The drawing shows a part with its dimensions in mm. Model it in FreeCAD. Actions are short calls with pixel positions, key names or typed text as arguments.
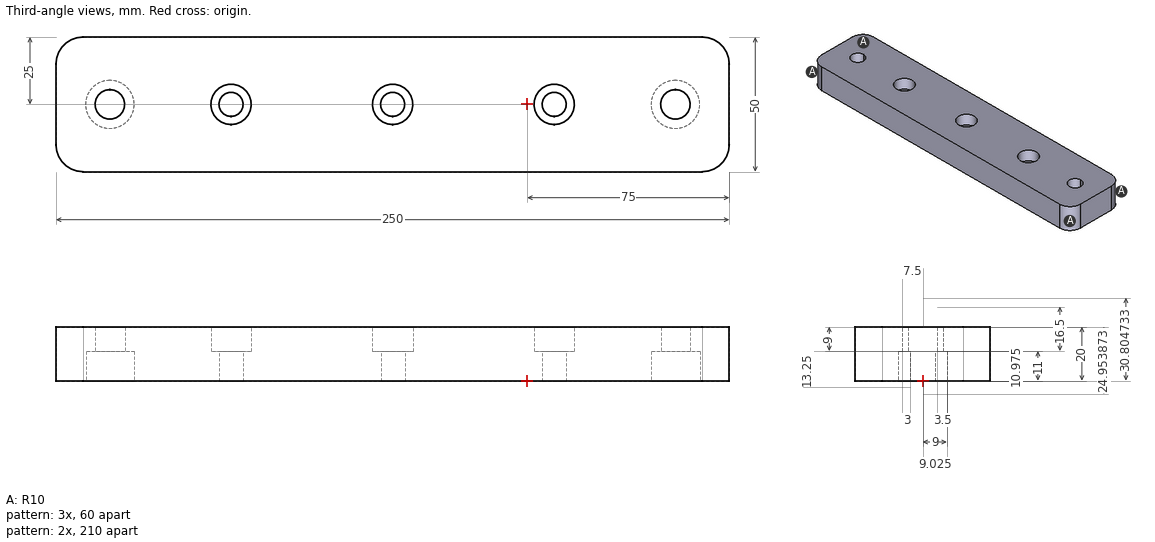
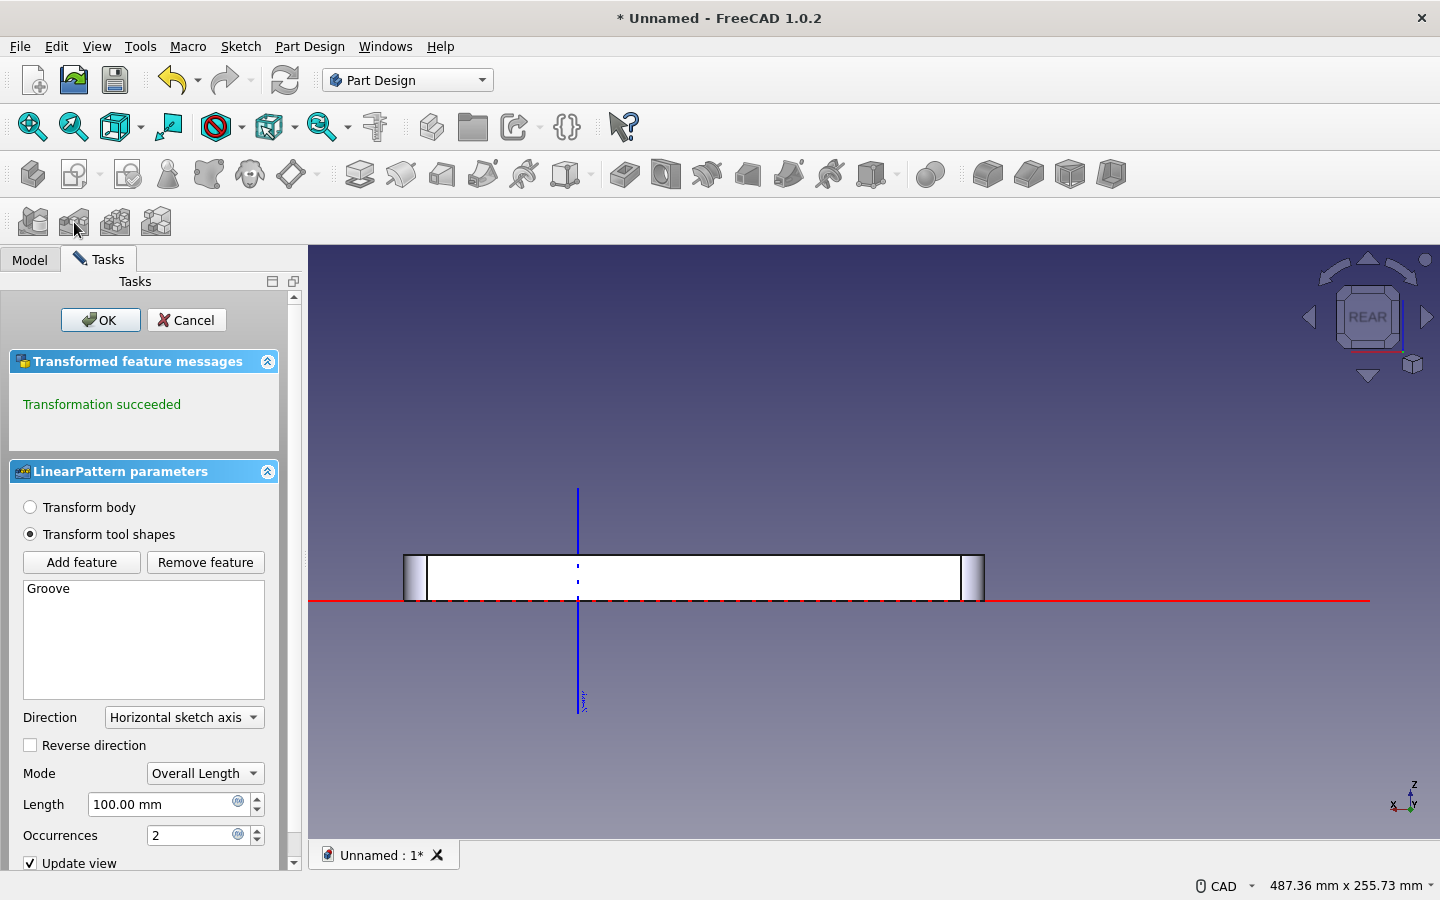
click(185, 718)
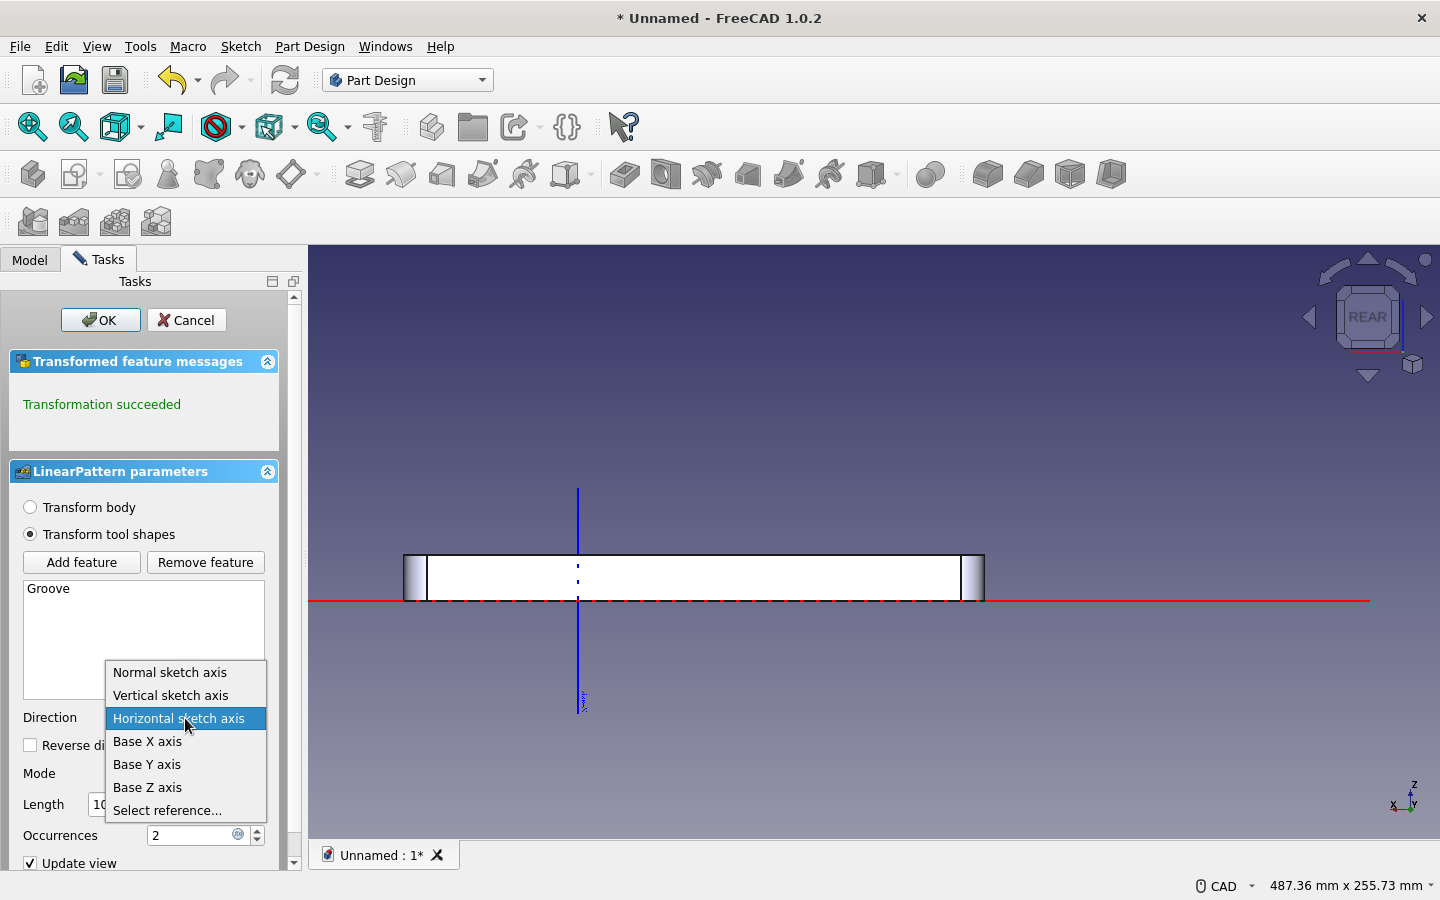
click(184, 742)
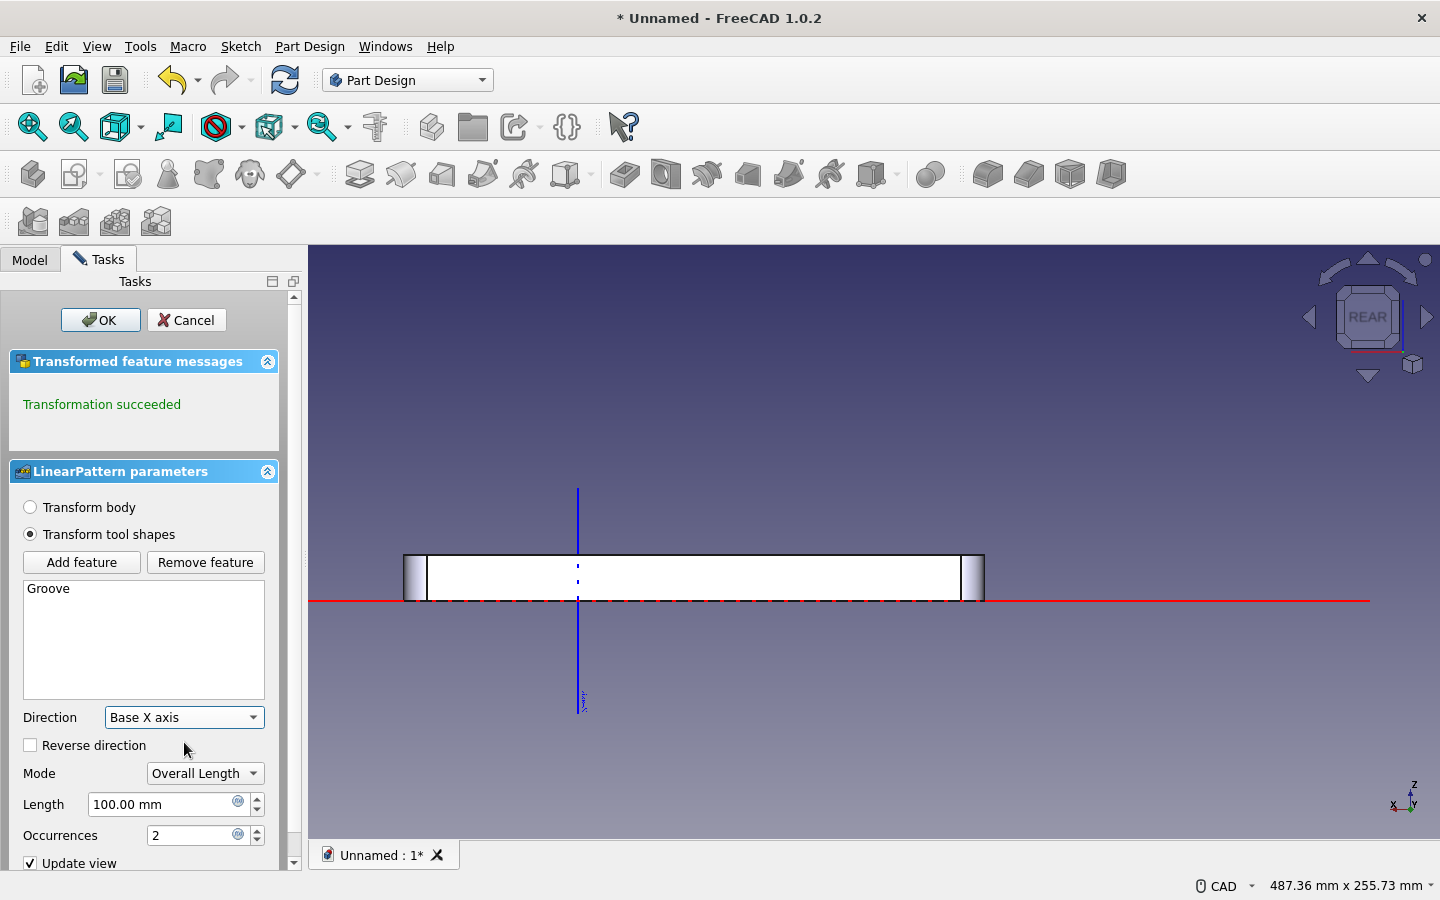
click(206, 774)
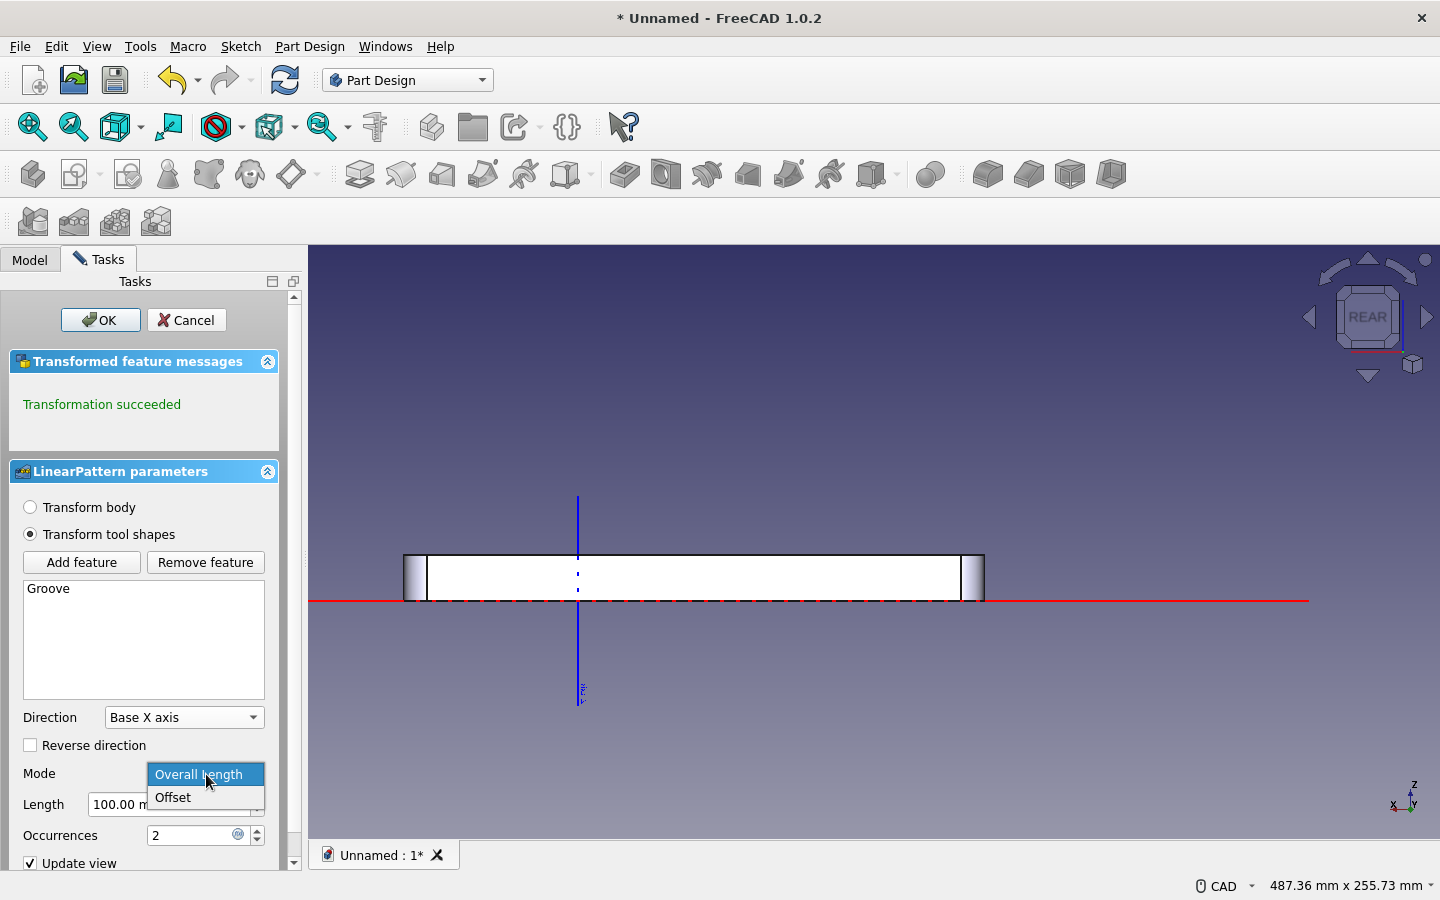
click(204, 798)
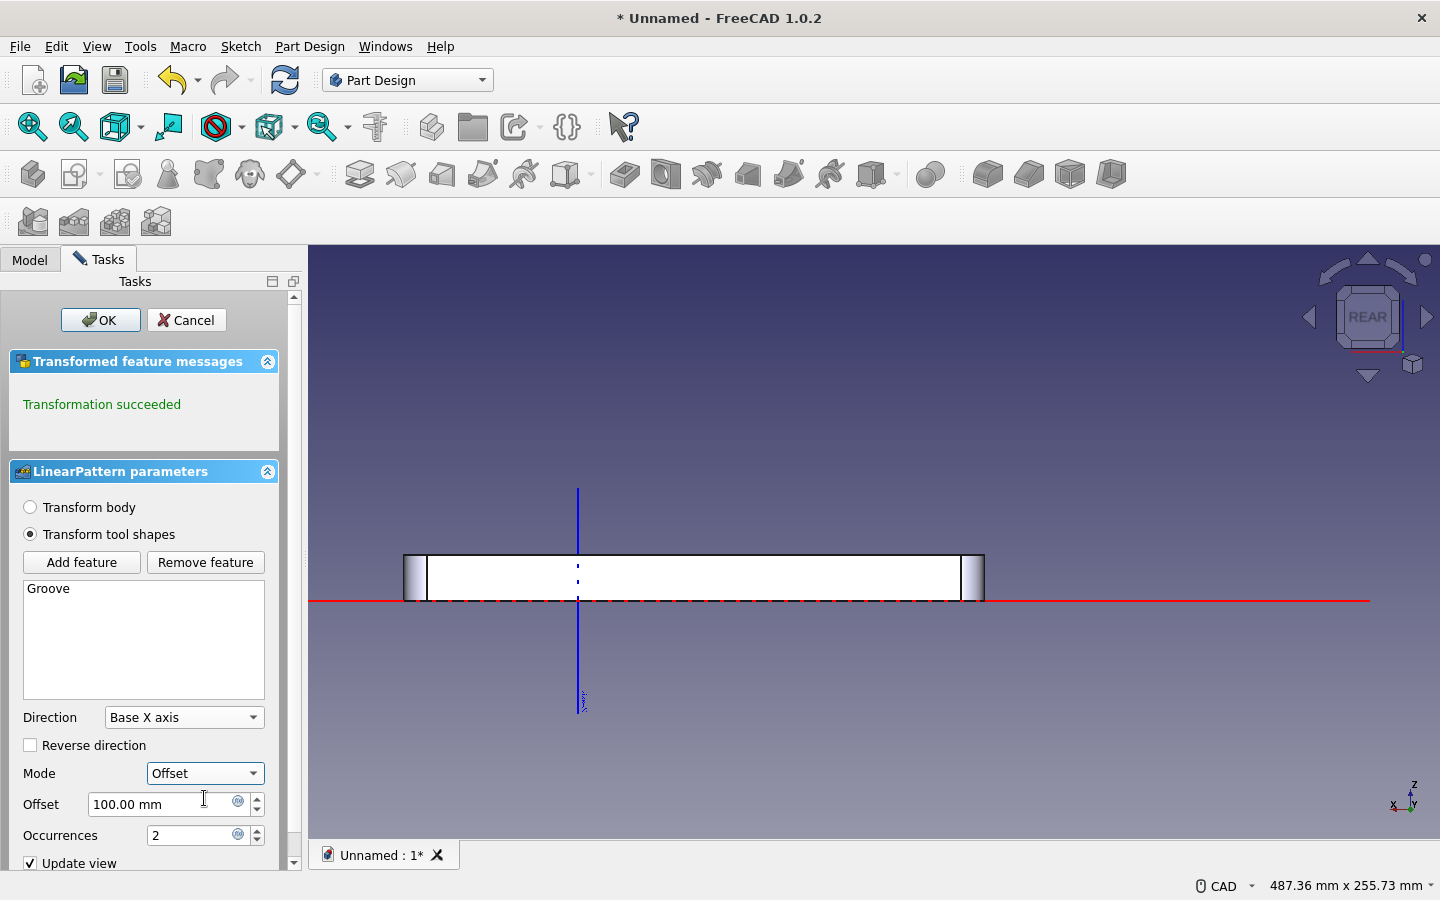
triple_click(170, 804)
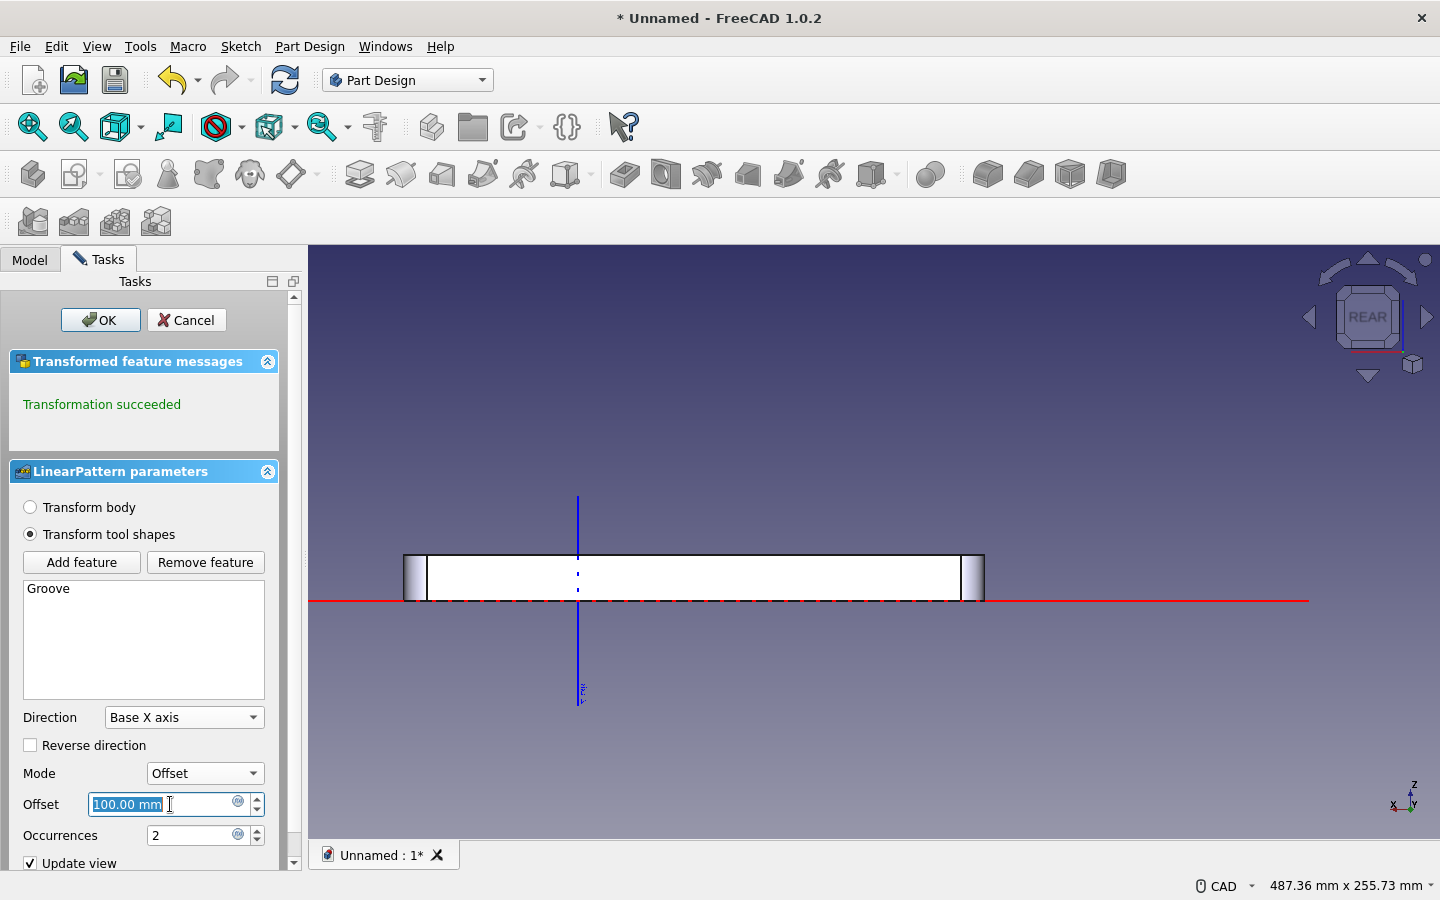
text(60)
key(Tab)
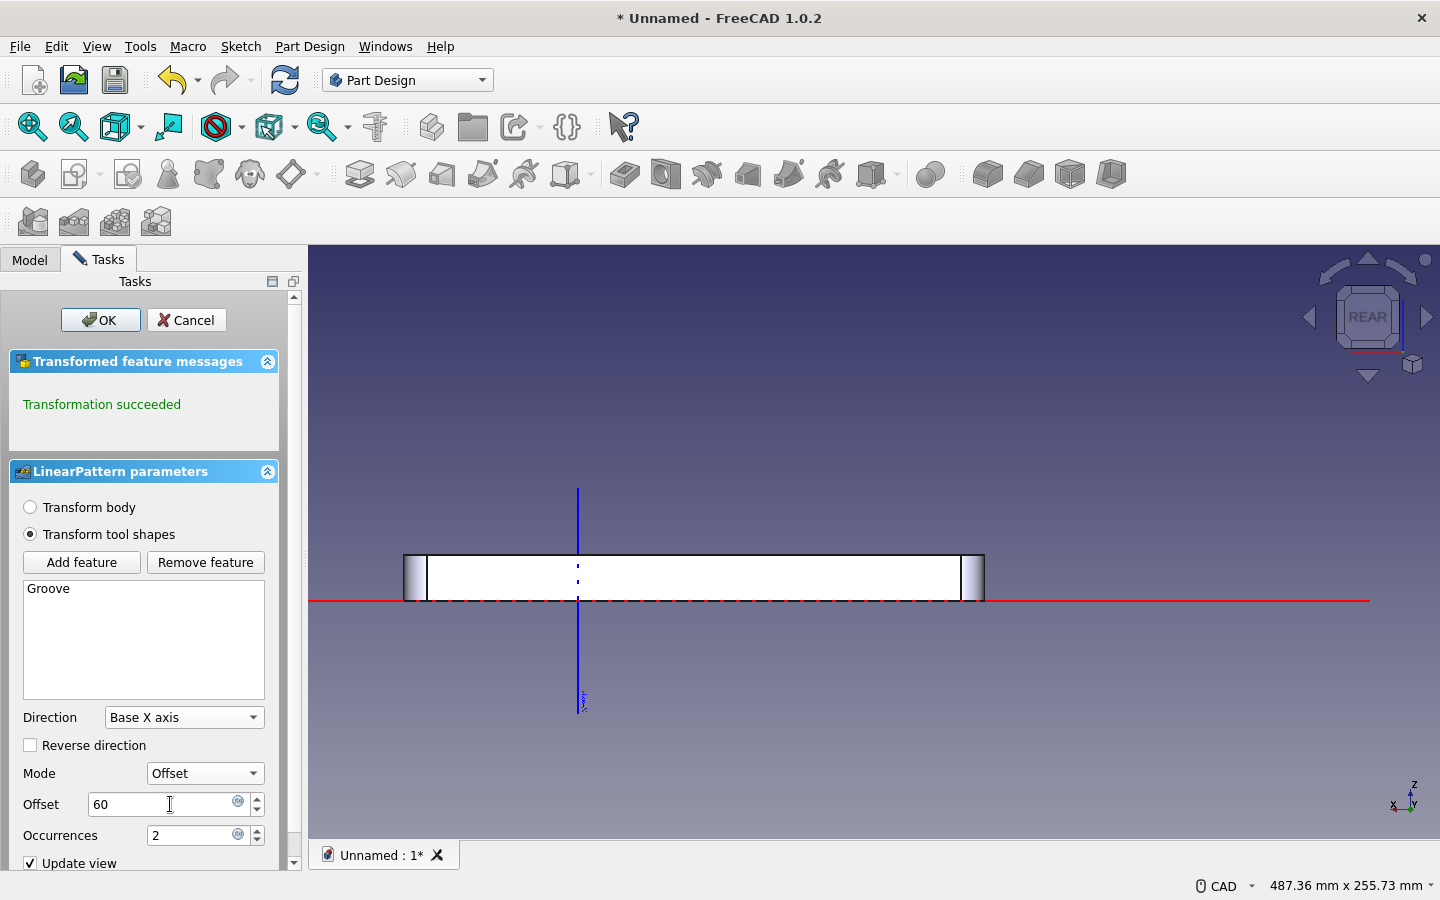
triple_click(199, 836)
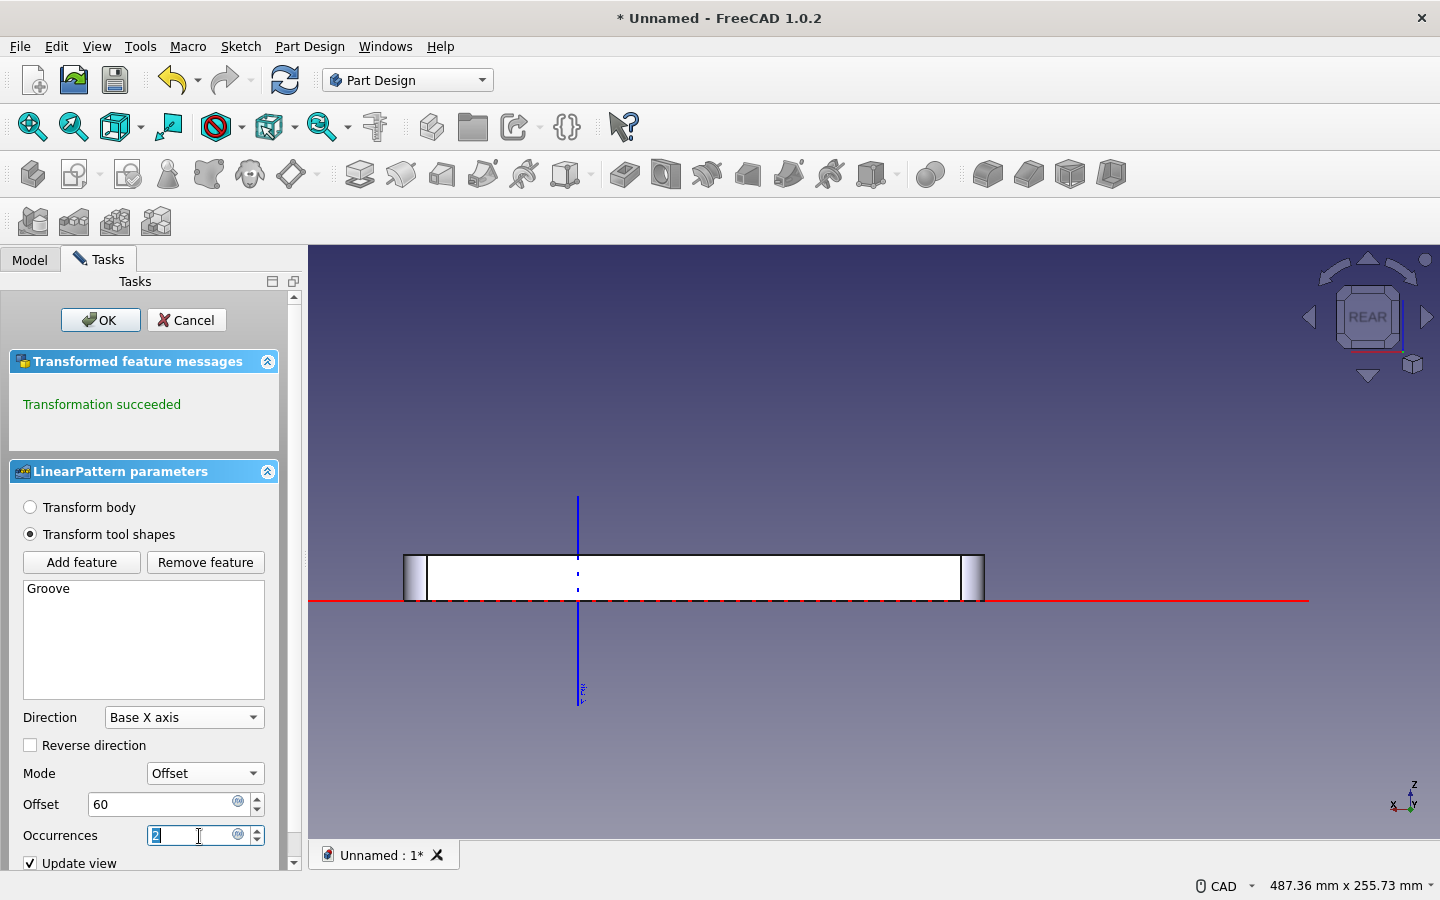
text(3)
key(Tab)